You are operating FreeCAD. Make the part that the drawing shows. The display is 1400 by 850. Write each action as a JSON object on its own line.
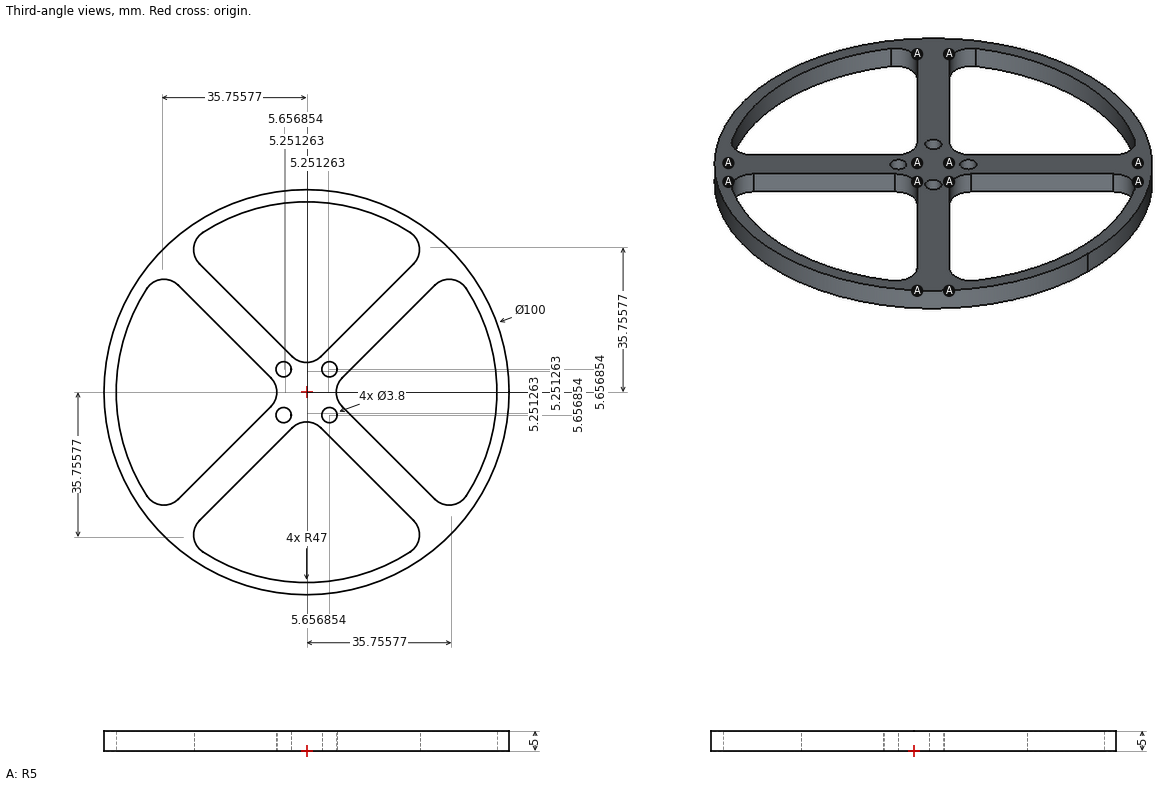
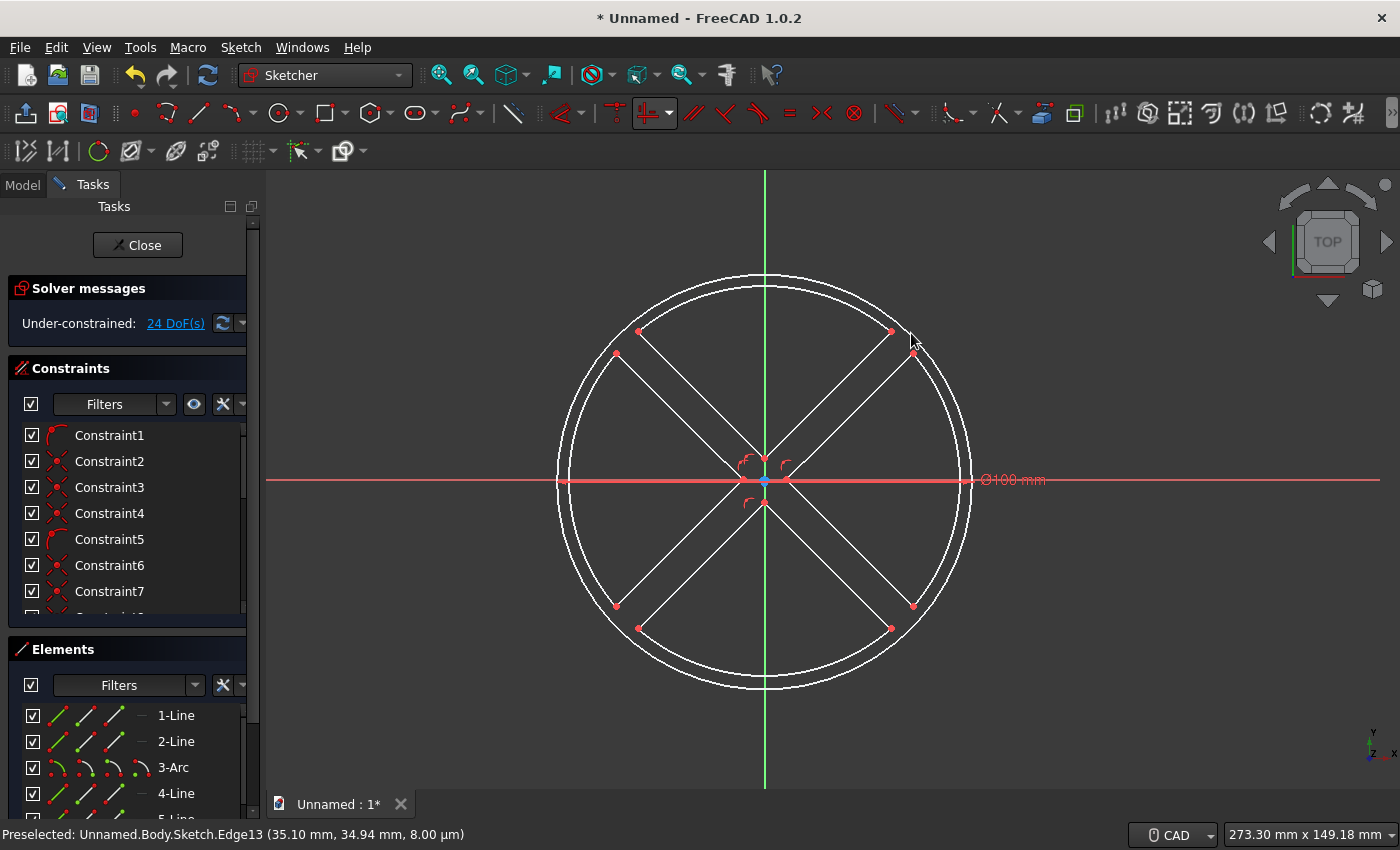
{"action": "left_click", "coordinate": [911, 335]}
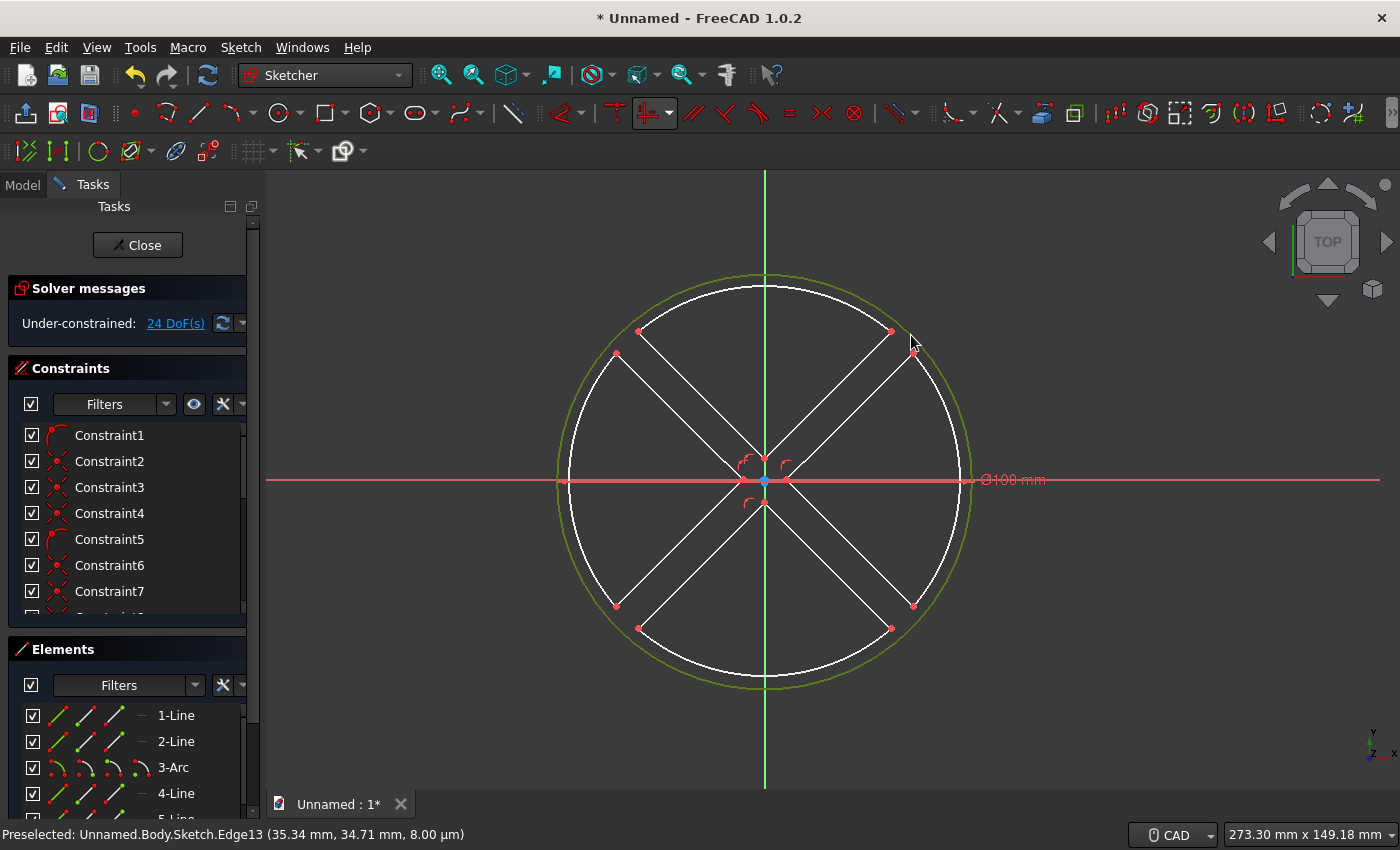
{"action": "left_click", "coordinate": [952, 535]}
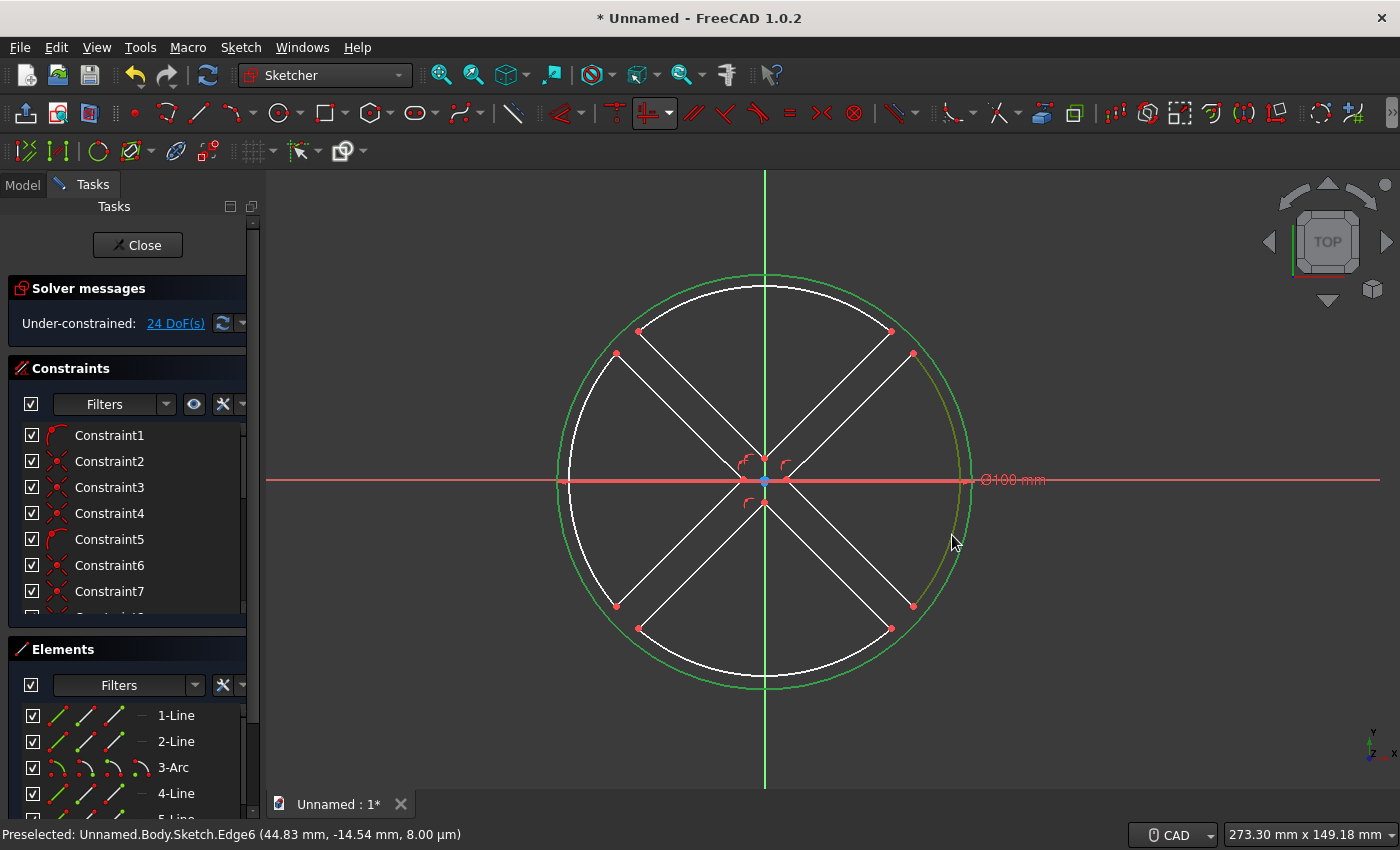
{"action": "left_click", "coordinate": [616, 114]}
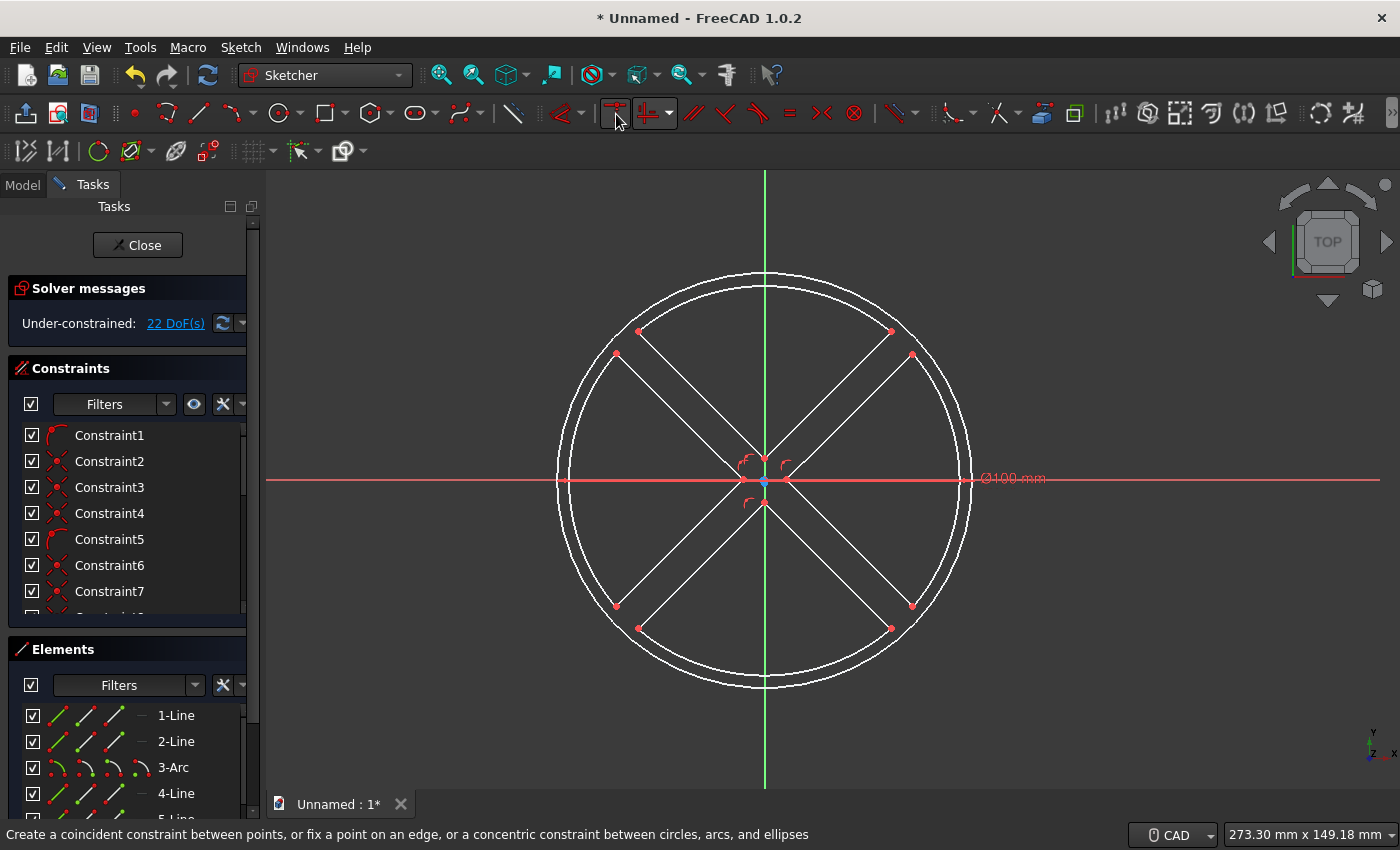
{"action": "left_click", "coordinate": [911, 333]}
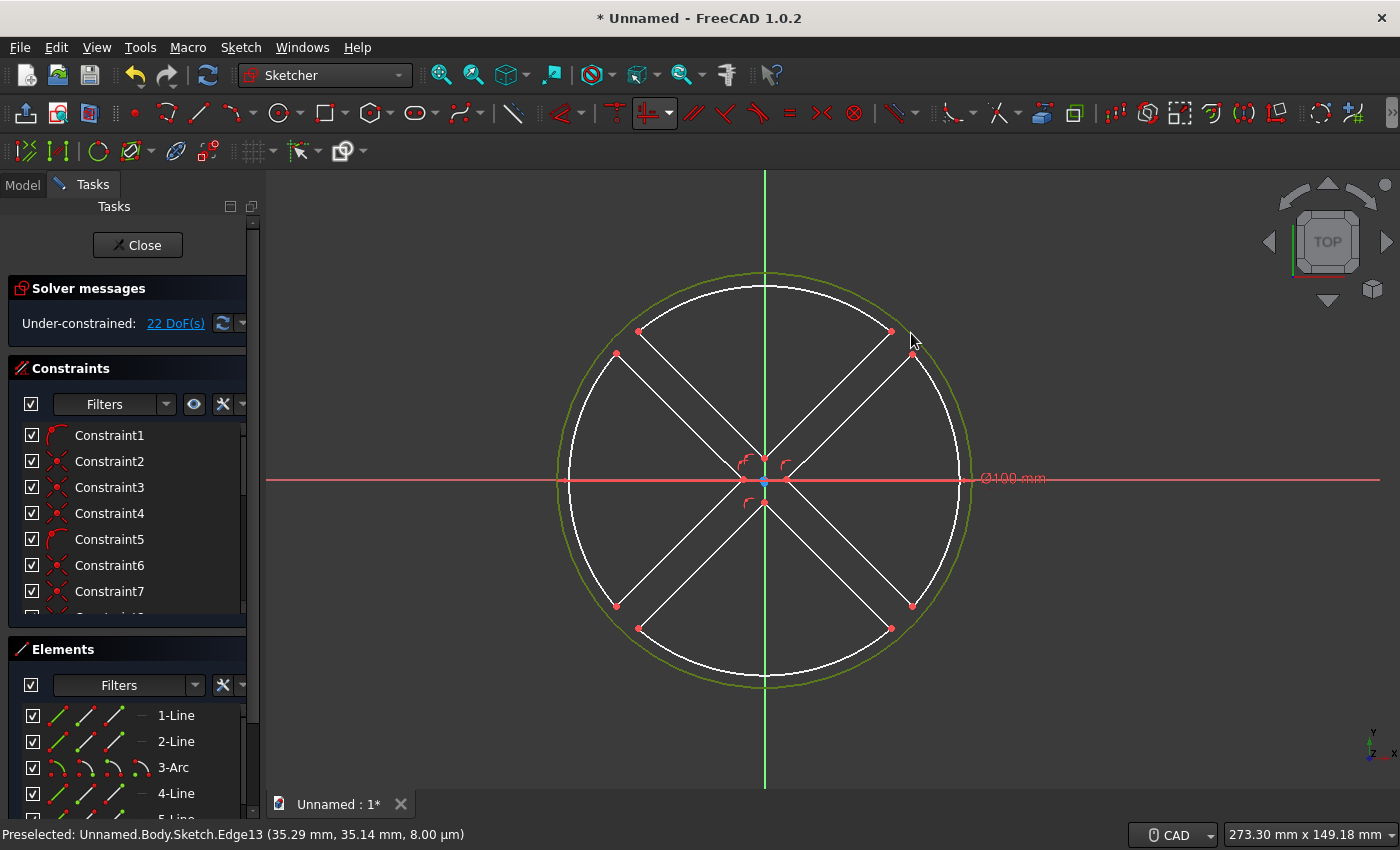
{"action": "left_click", "coordinate": [577, 426]}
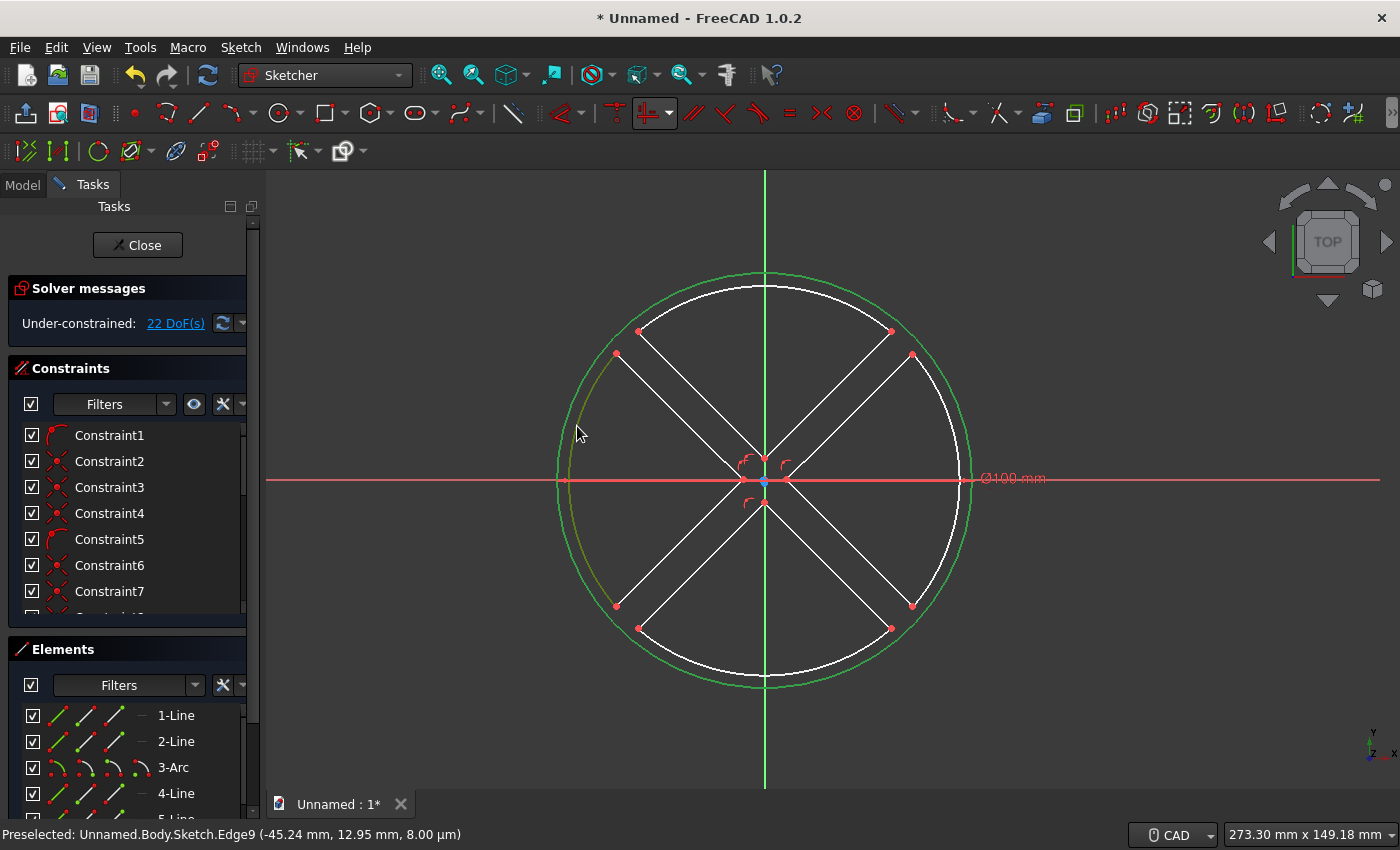
{"action": "left_click", "coordinate": [616, 114]}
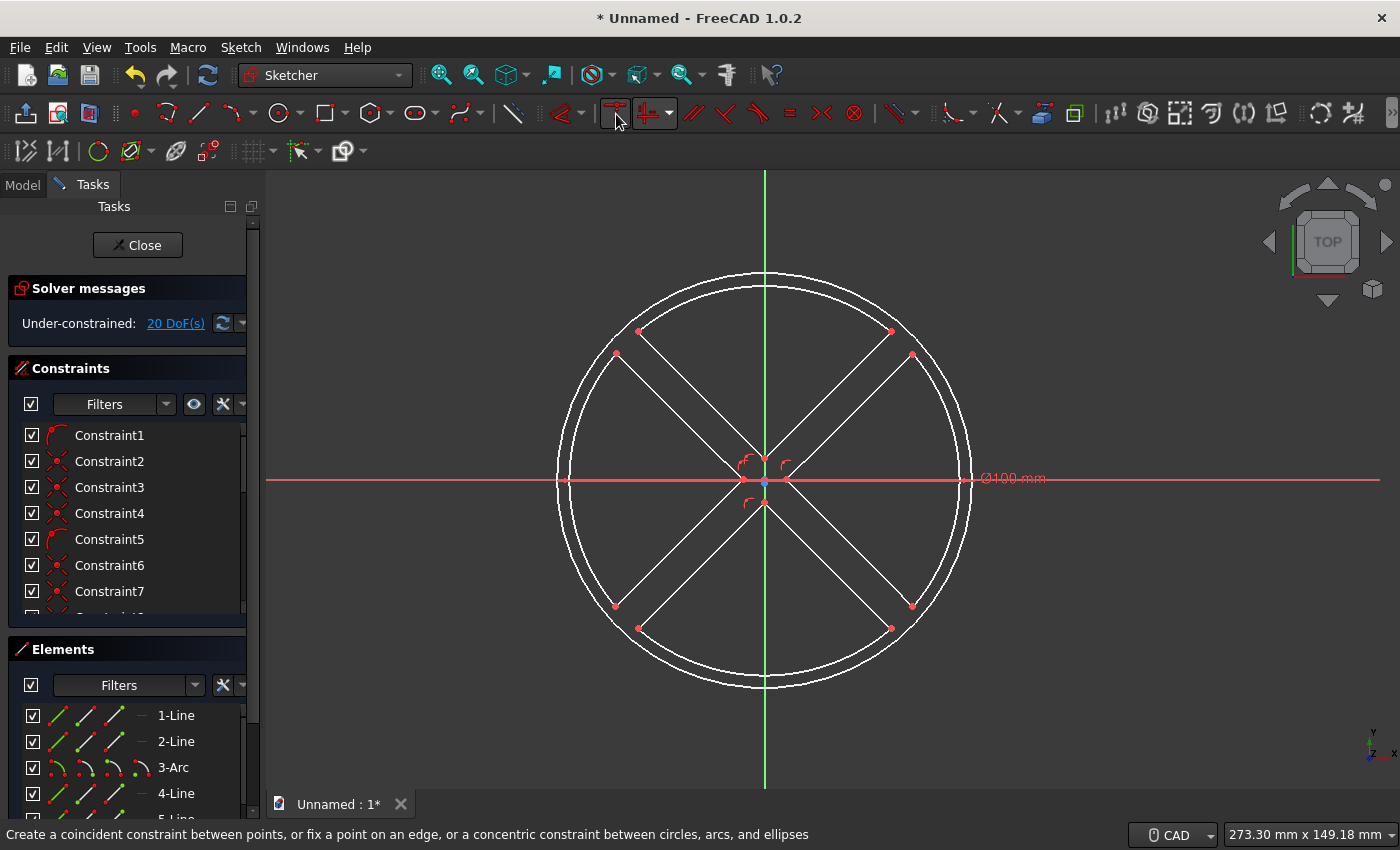
{"action": "left_click", "coordinate": [911, 333]}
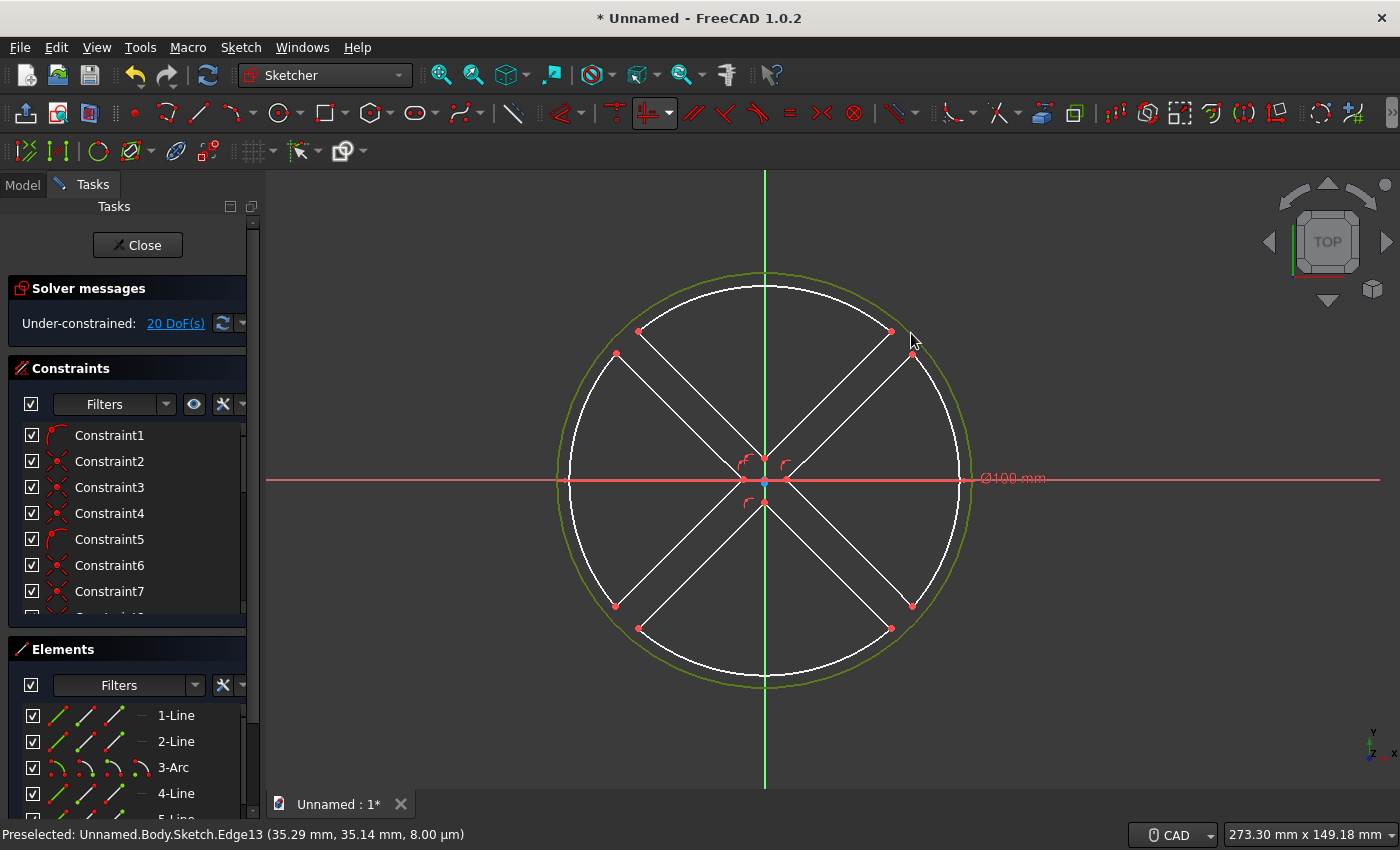
{"action": "left_click", "coordinate": [819, 294]}